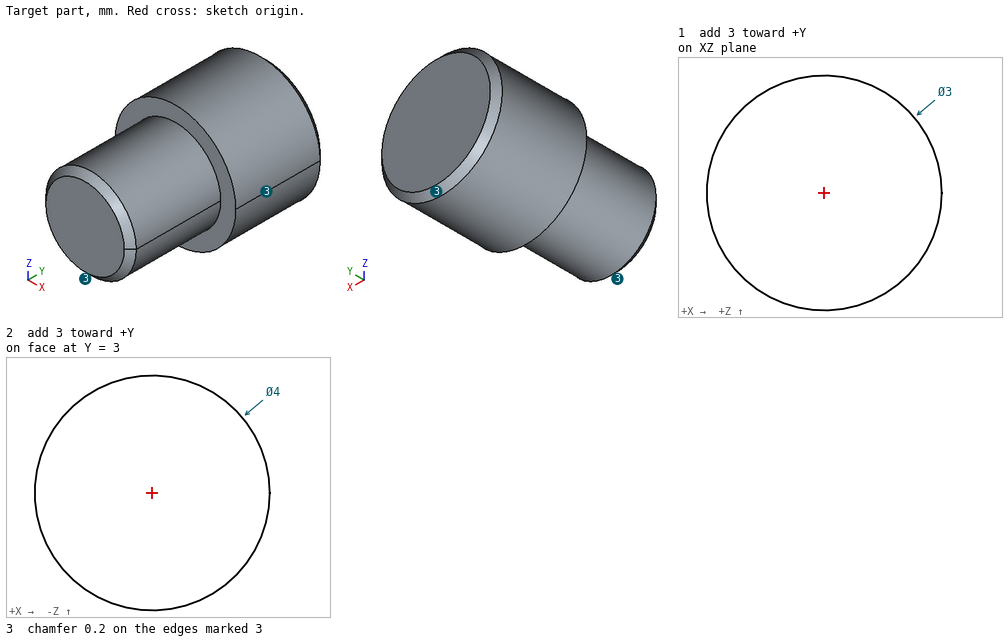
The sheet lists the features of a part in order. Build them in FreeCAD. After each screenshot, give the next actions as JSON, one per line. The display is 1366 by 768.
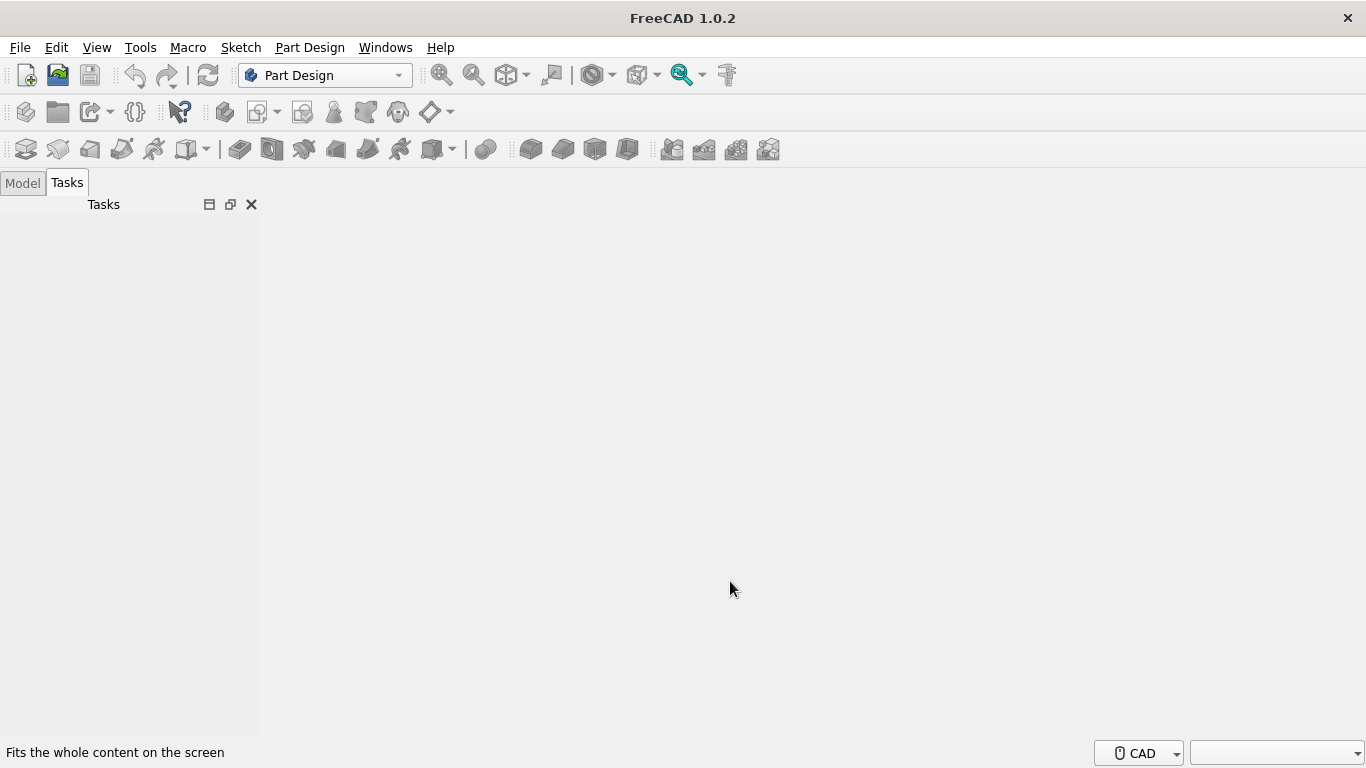
{"action": "key", "text": "ctrl+n"}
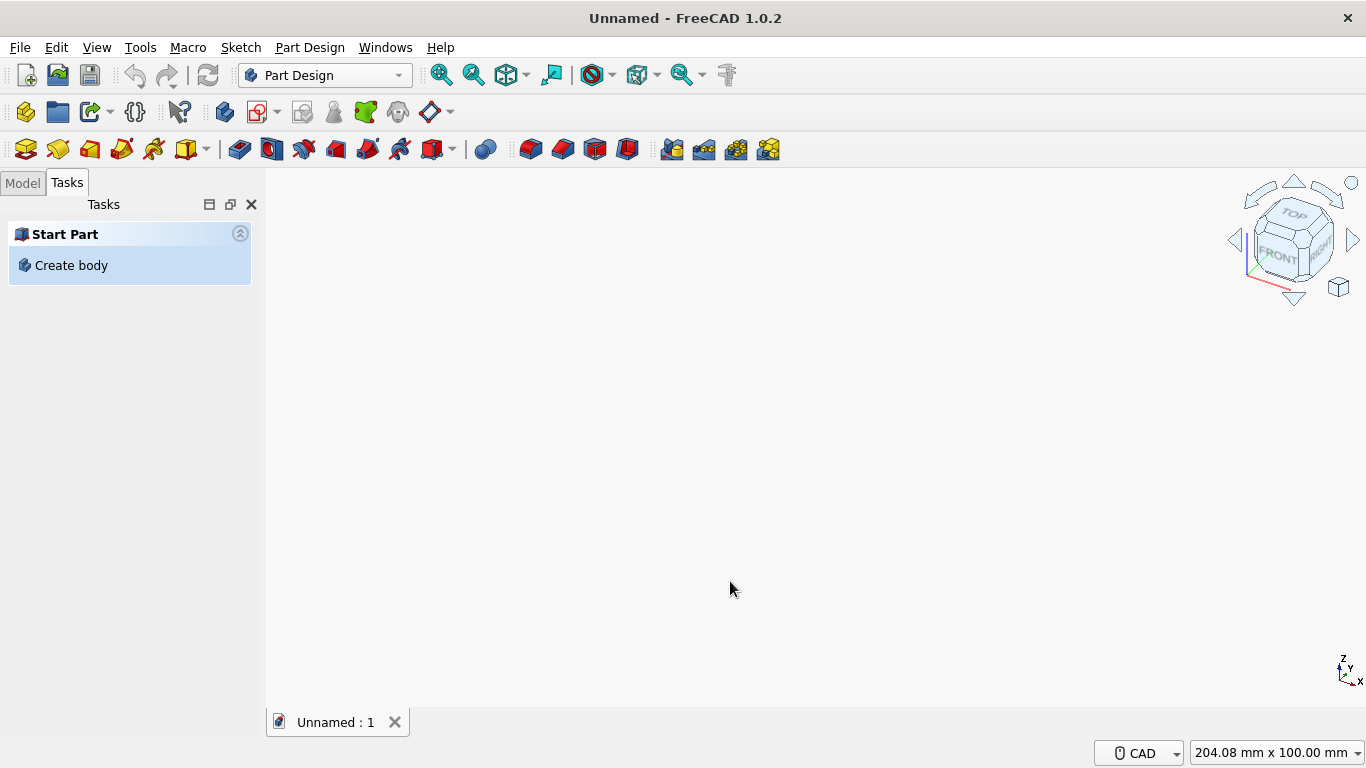
{"action": "left_click", "coordinate": [258, 112]}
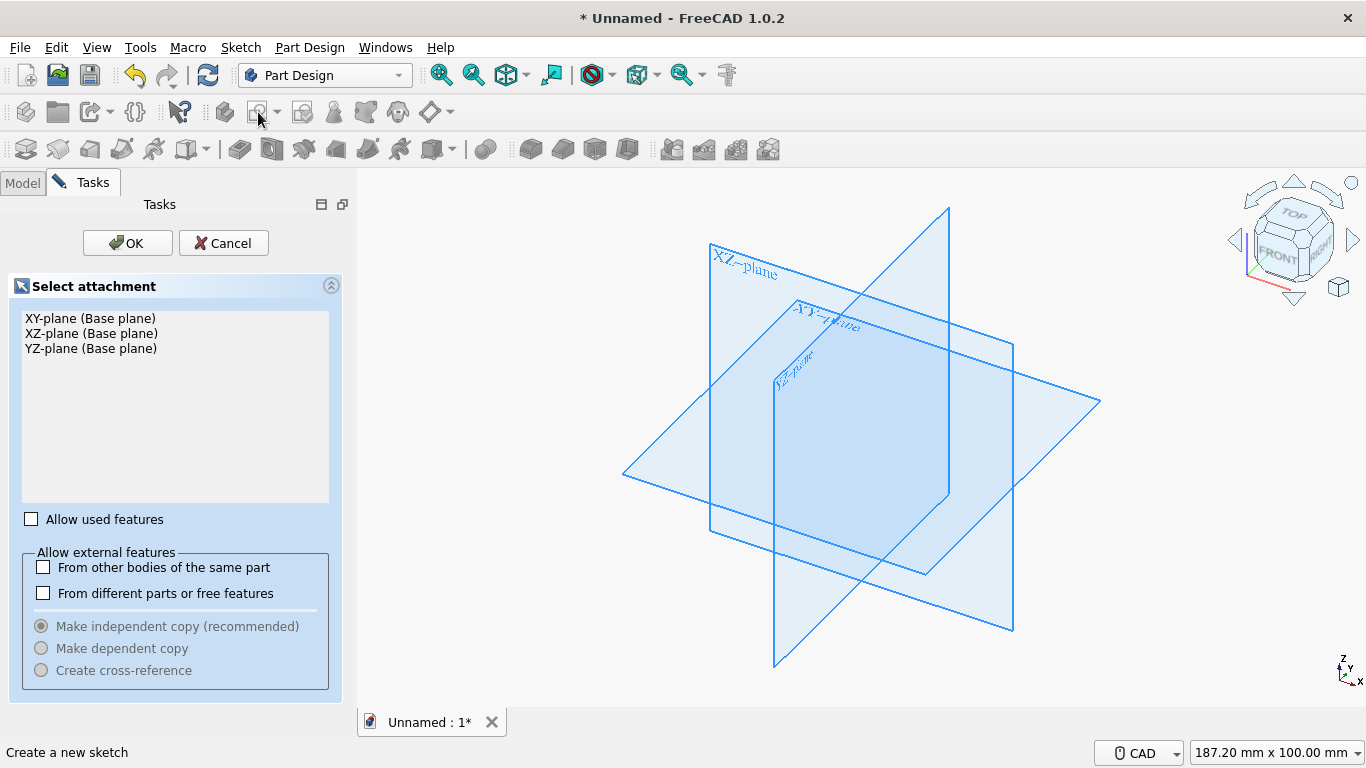
{"action": "left_click", "coordinate": [82, 334]}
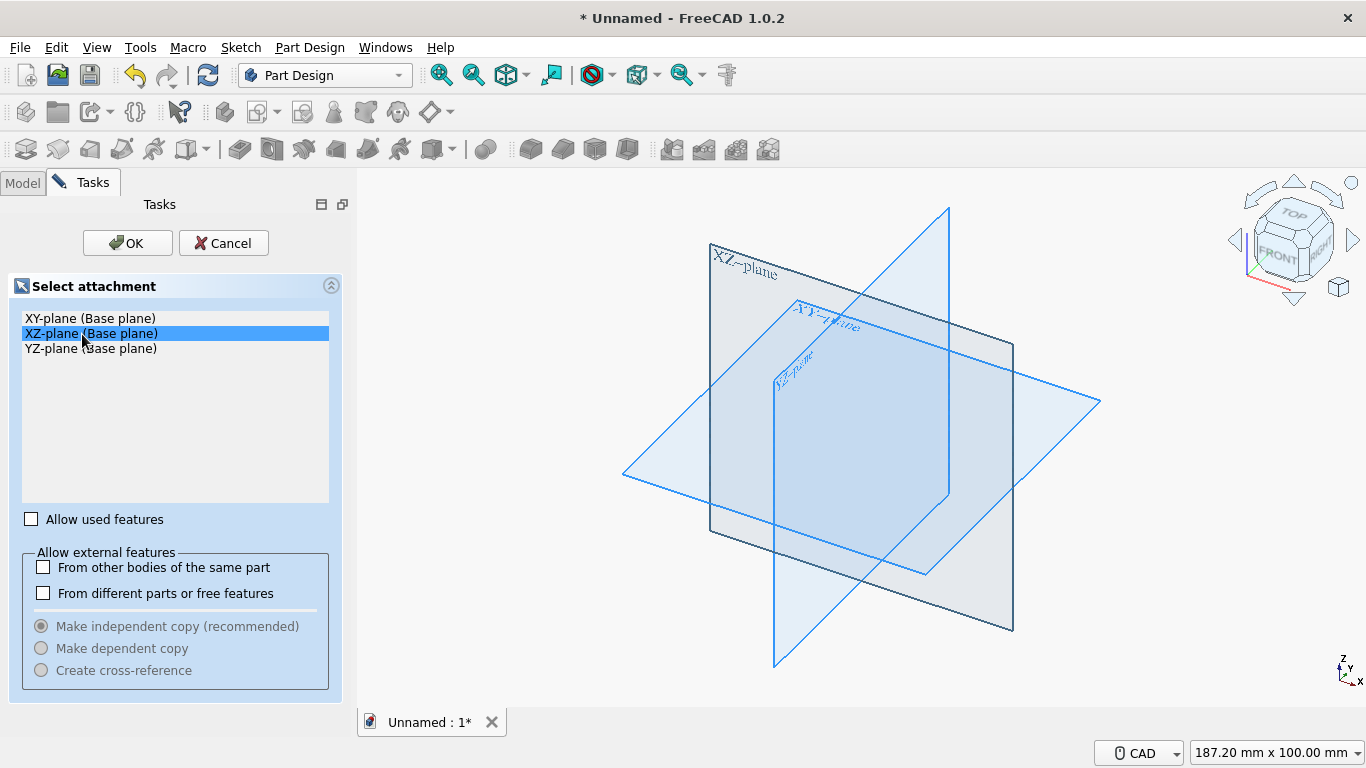
{"action": "left_click", "coordinate": [128, 243]}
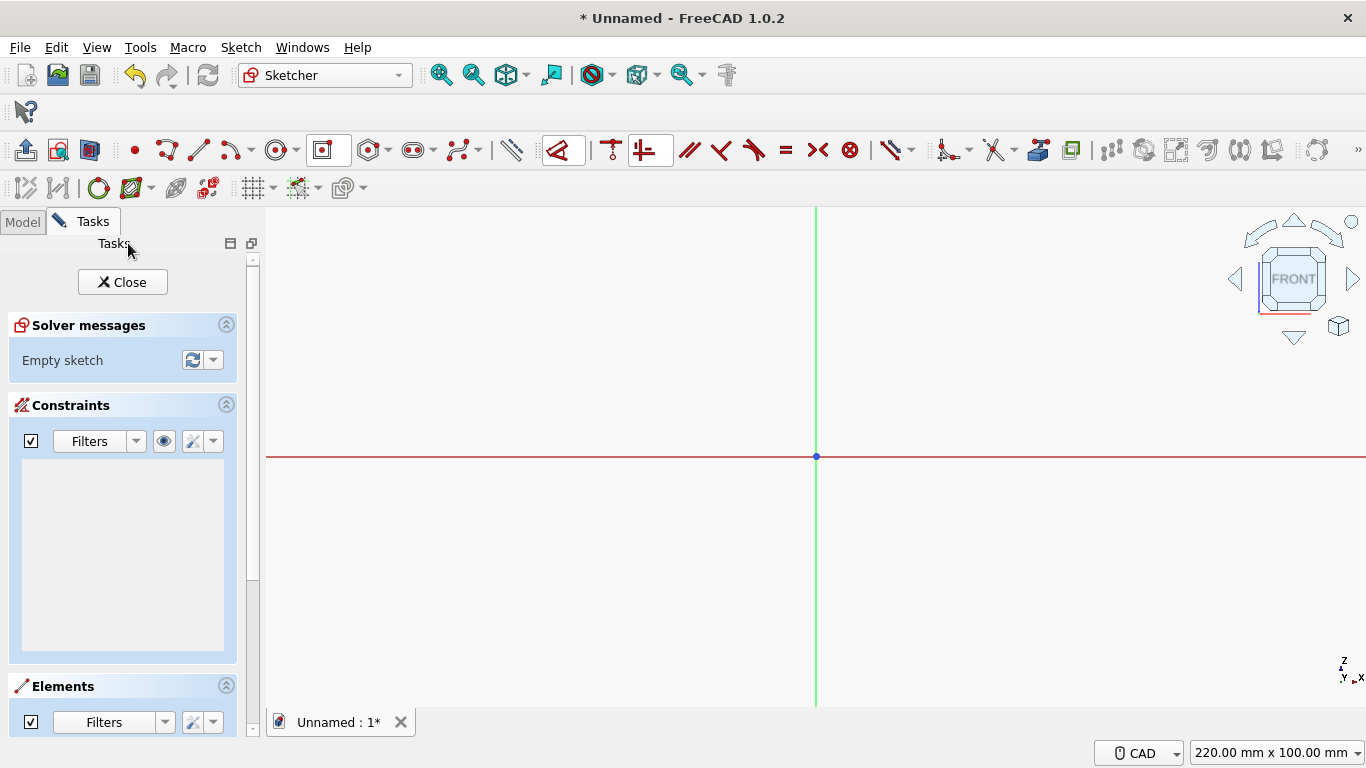
{"action": "scroll", "coordinate": [820, 457], "scroll_direction": "up", "scroll_amount": 15}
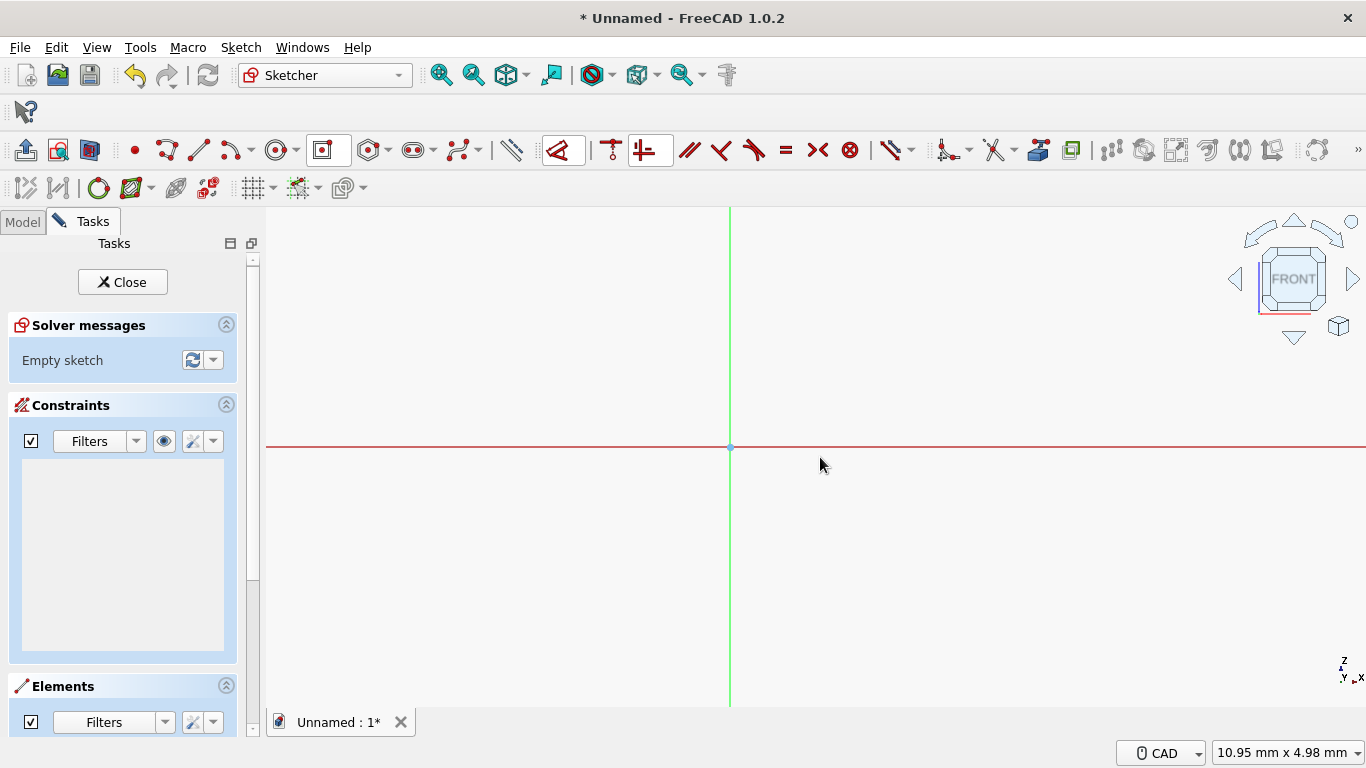
{"action": "key", "text": "g c"}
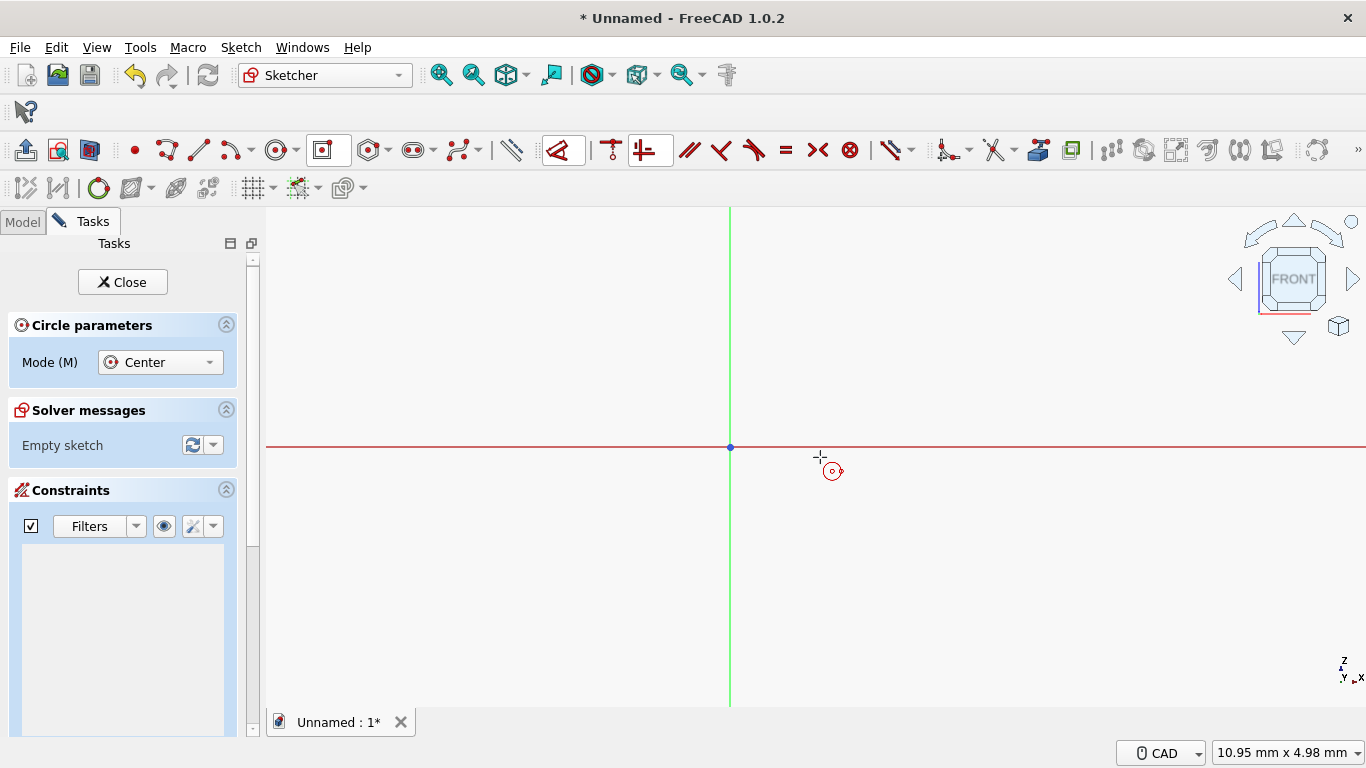
{"action": "left_click", "coordinate": [730, 447]}
{"action": "mouse_move", "coordinate": [837, 341]}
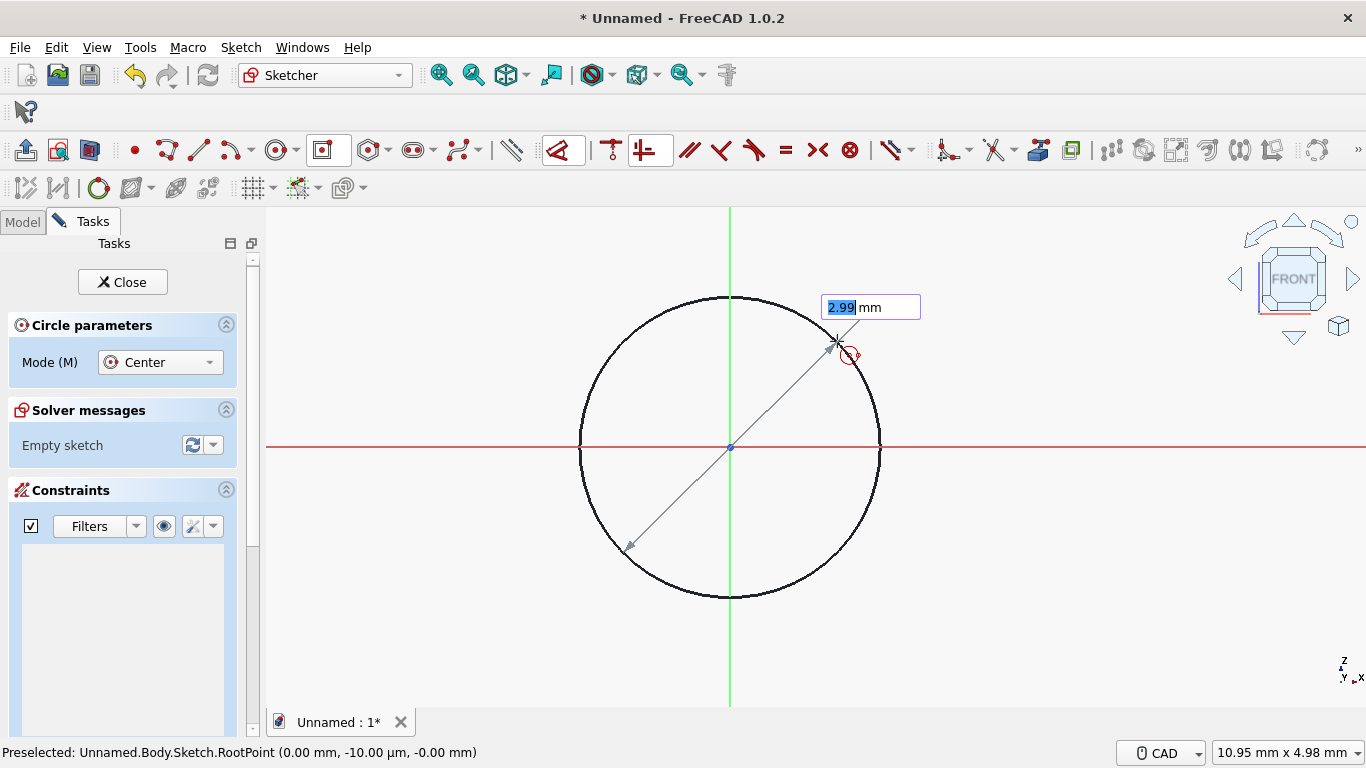
{"action": "type", "text": "3"}
{"action": "key", "text": "Return"}
{"action": "key", "text": "Escape"}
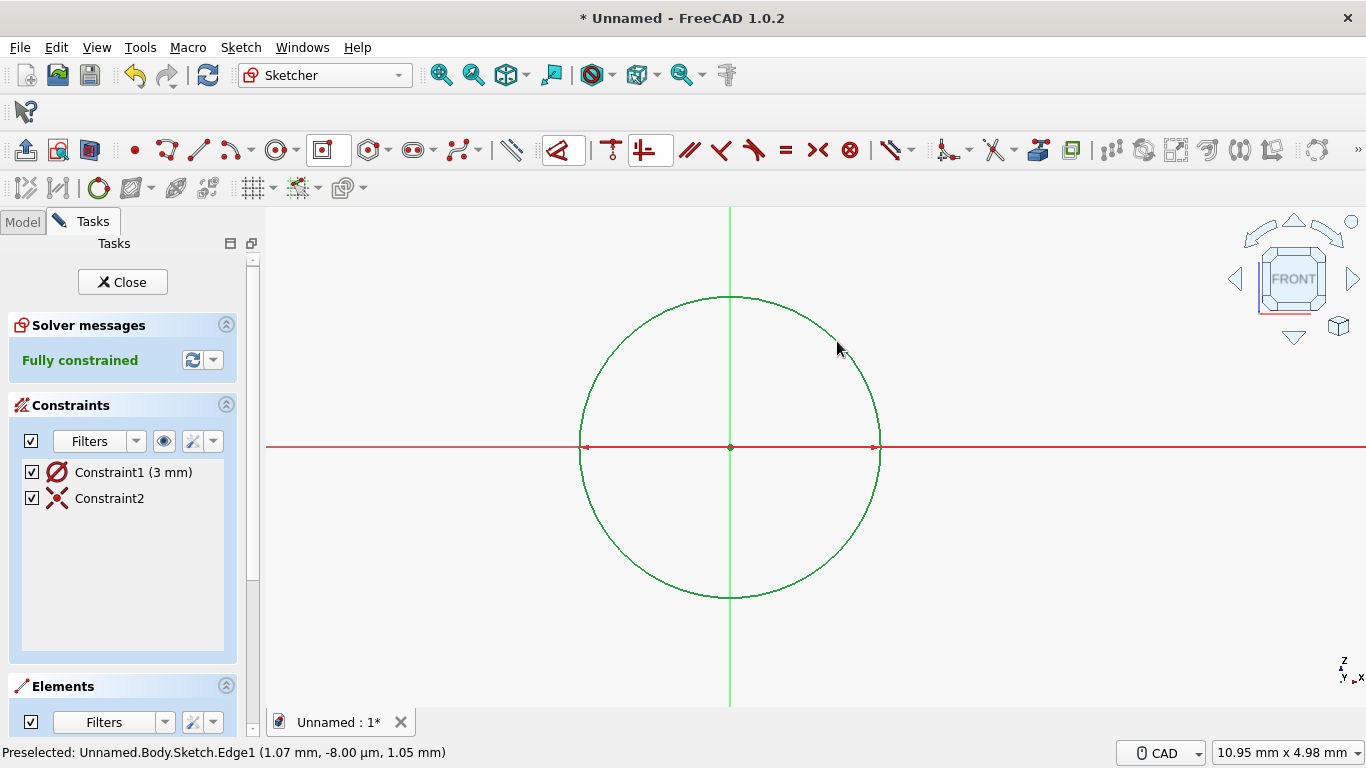
{"action": "left_click", "coordinate": [123, 282]}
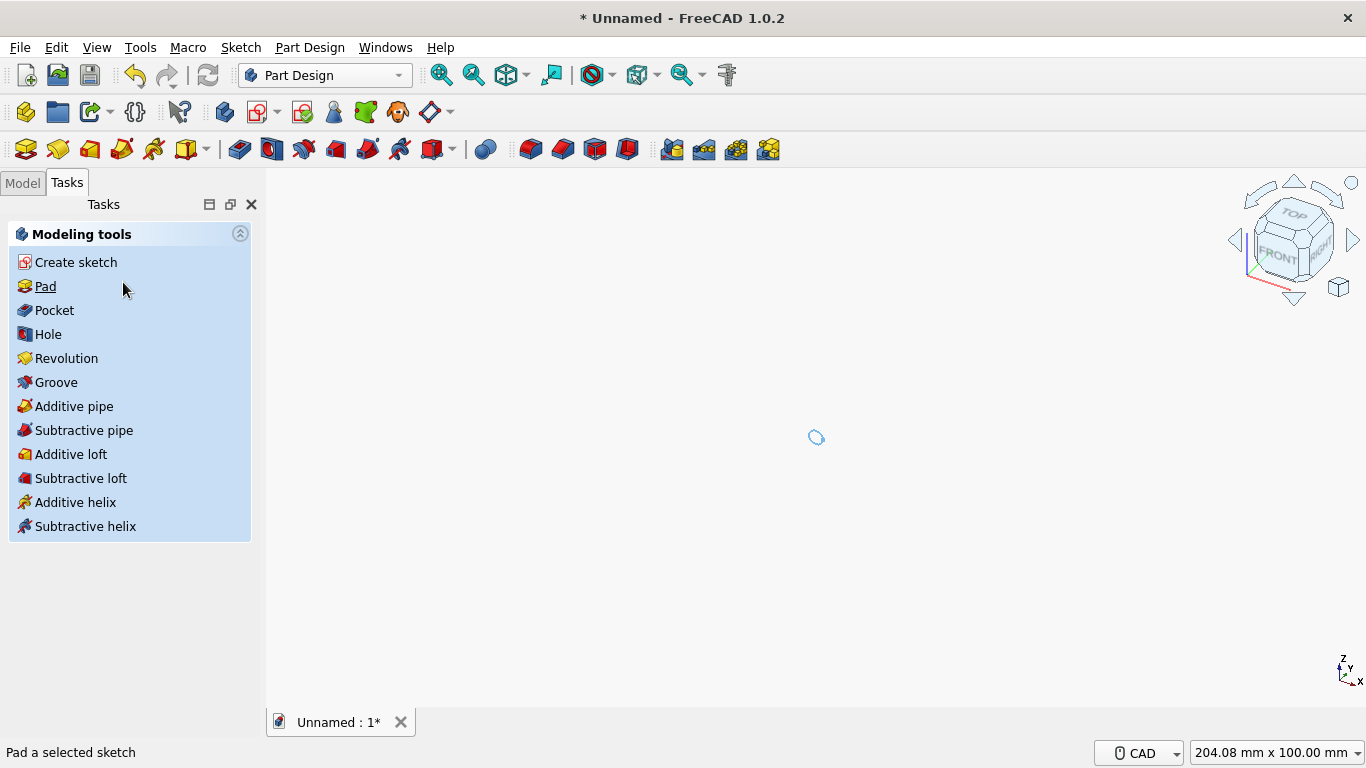
{"action": "left_click", "coordinate": [26, 150]}